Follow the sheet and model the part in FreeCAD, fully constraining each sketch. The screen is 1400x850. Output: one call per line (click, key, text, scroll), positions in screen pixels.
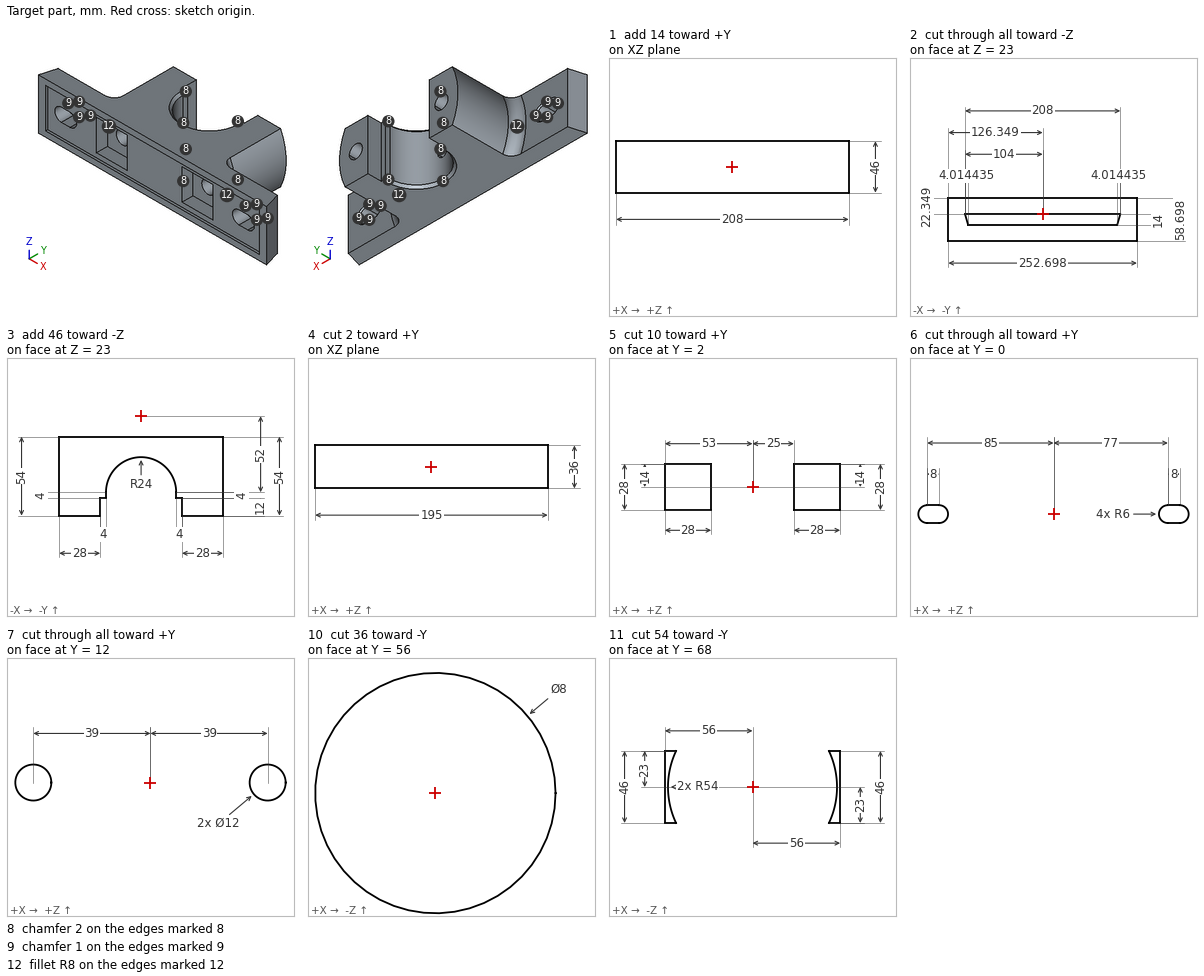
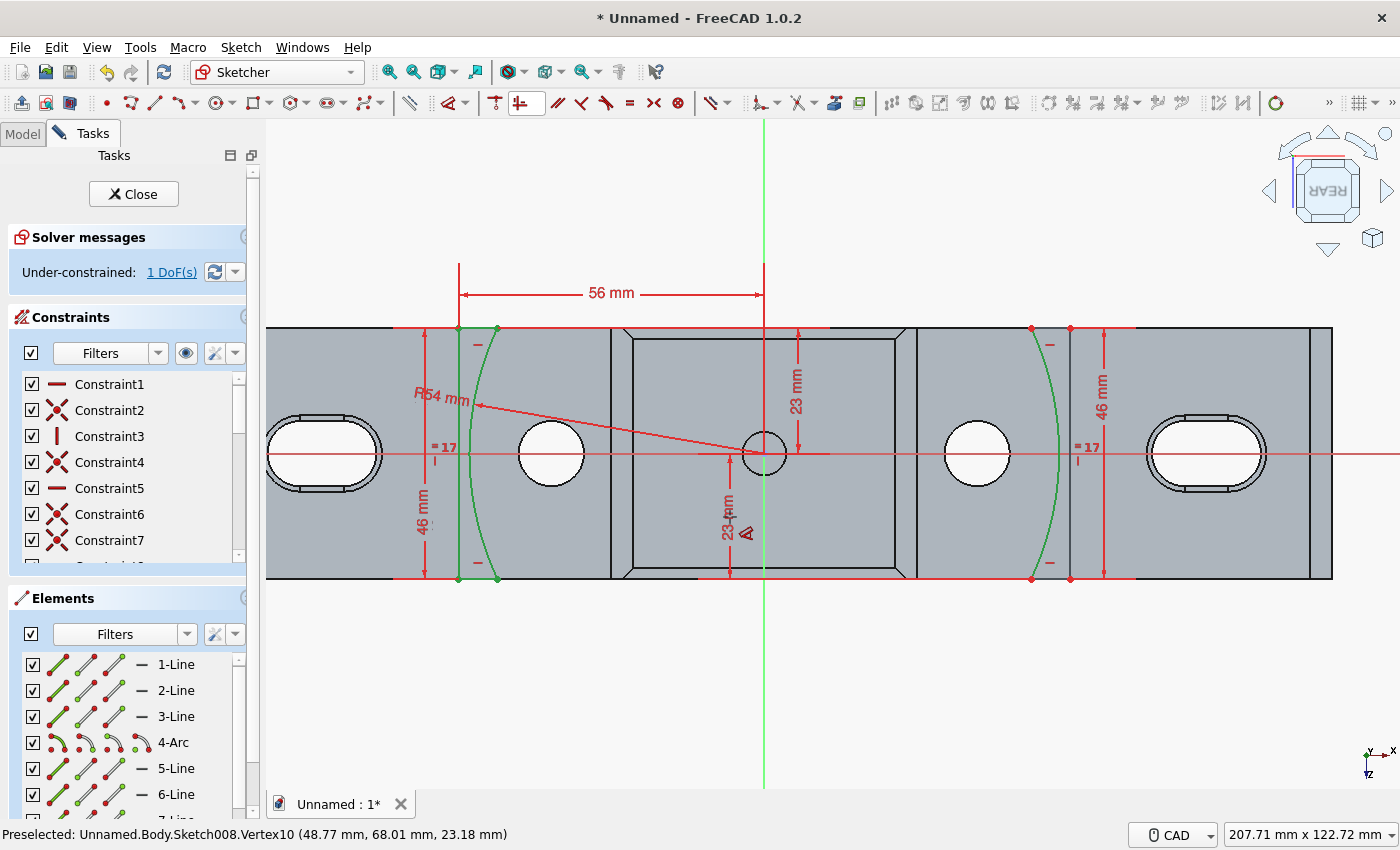
click(1070, 579)
click(917, 613)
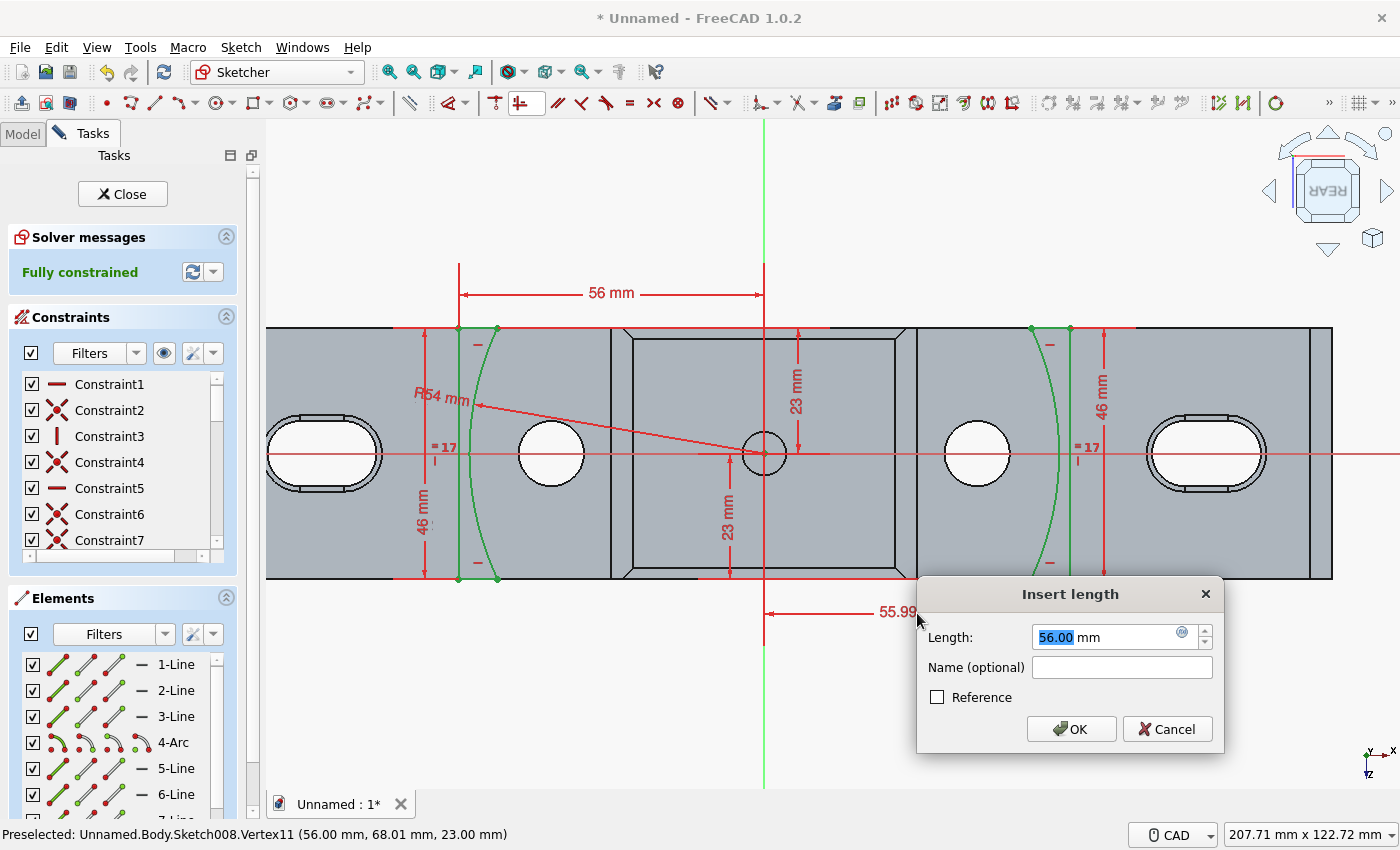
text(56)
key(Return)
key(Escape)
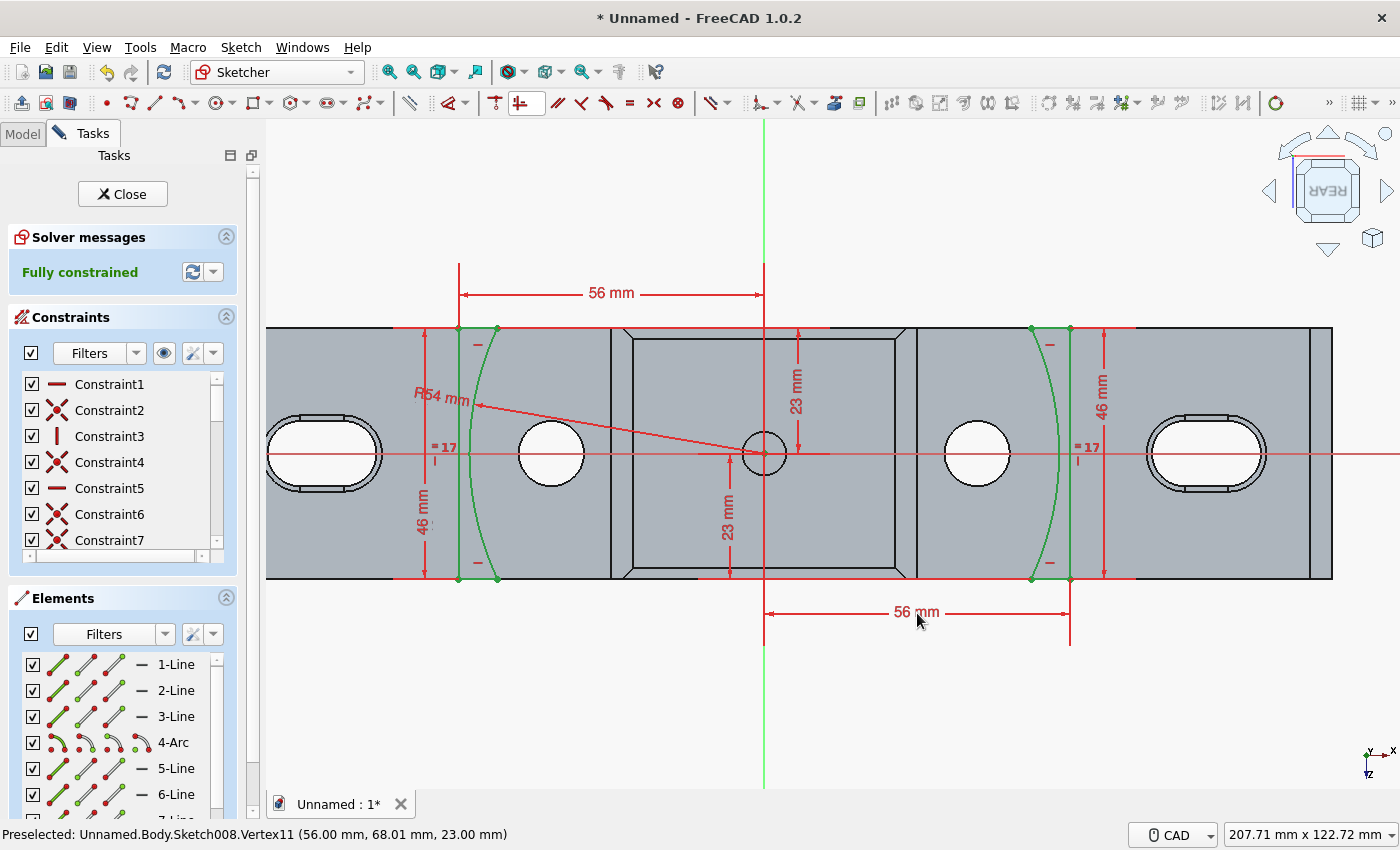
click(123, 194)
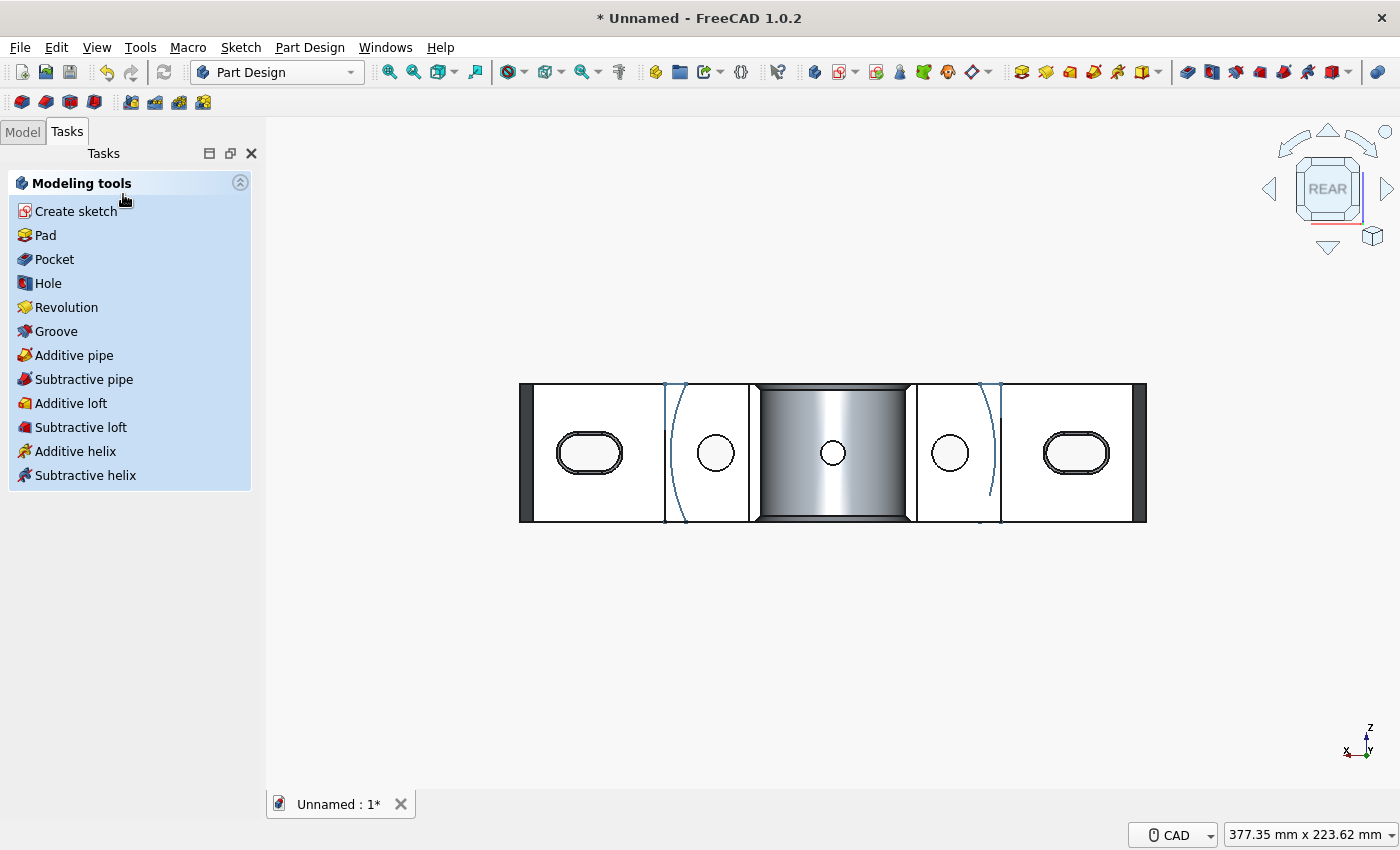
click(1188, 72)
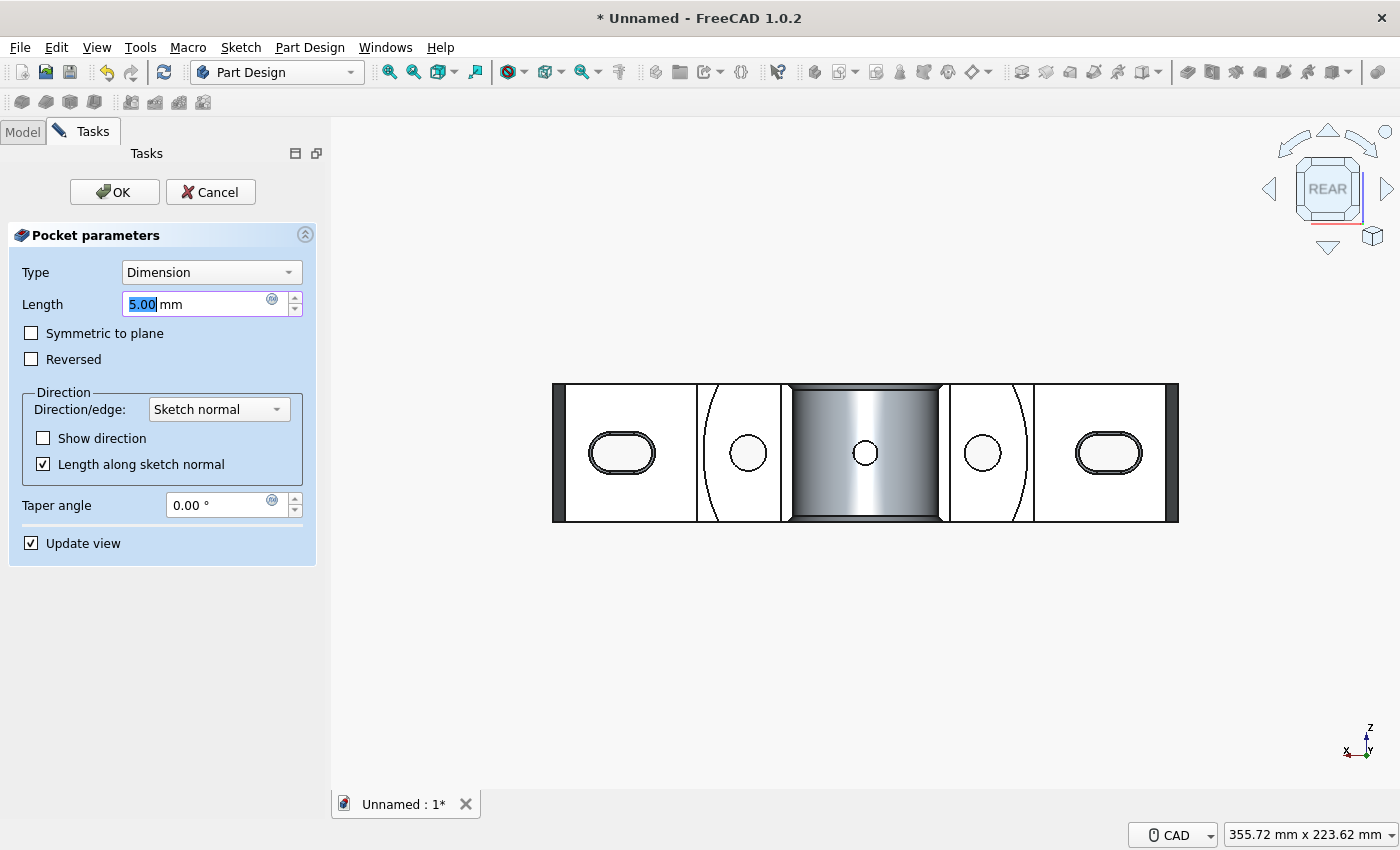
text(54)
key(Tab)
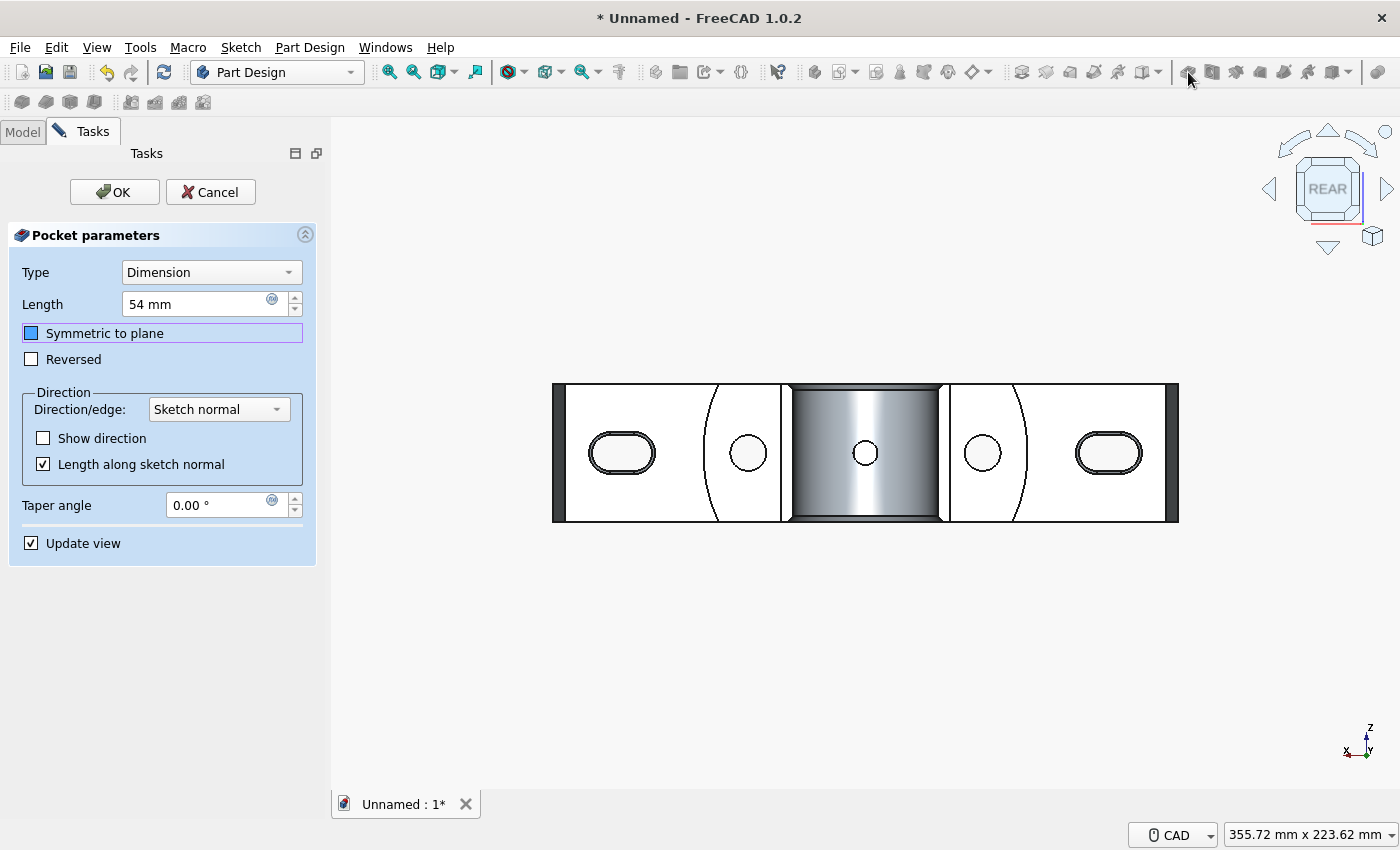
click(115, 192)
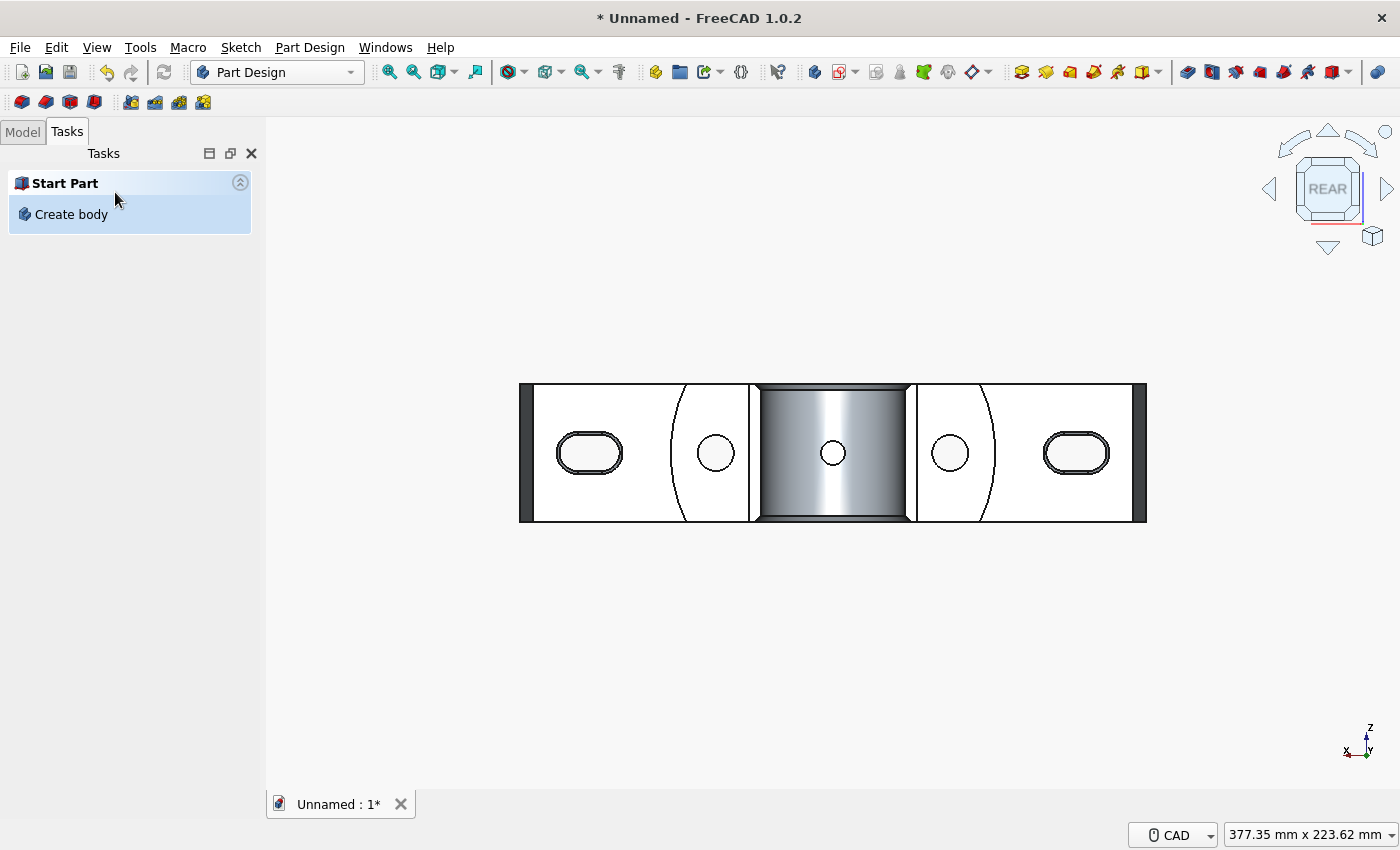
key(0)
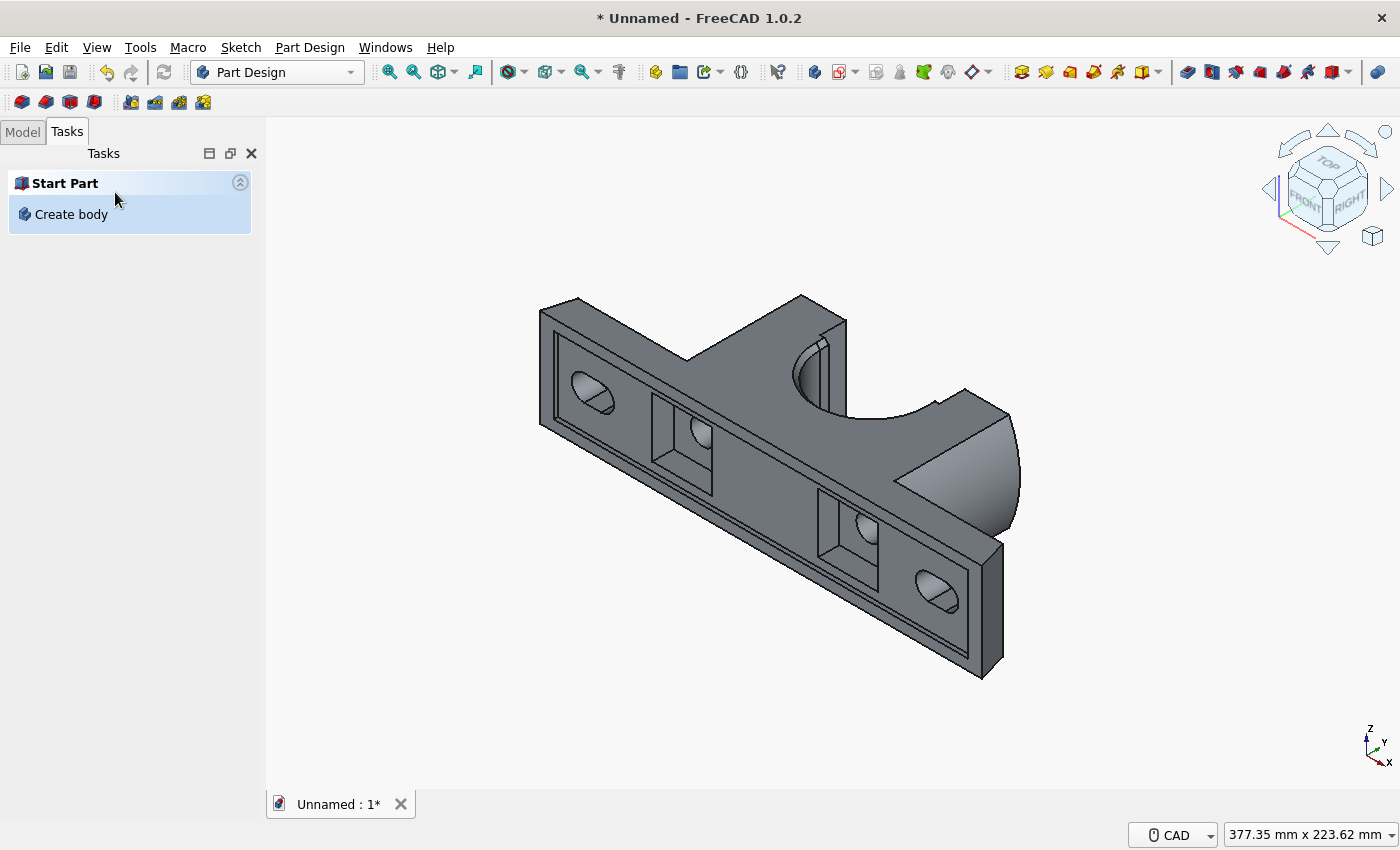
key(2)